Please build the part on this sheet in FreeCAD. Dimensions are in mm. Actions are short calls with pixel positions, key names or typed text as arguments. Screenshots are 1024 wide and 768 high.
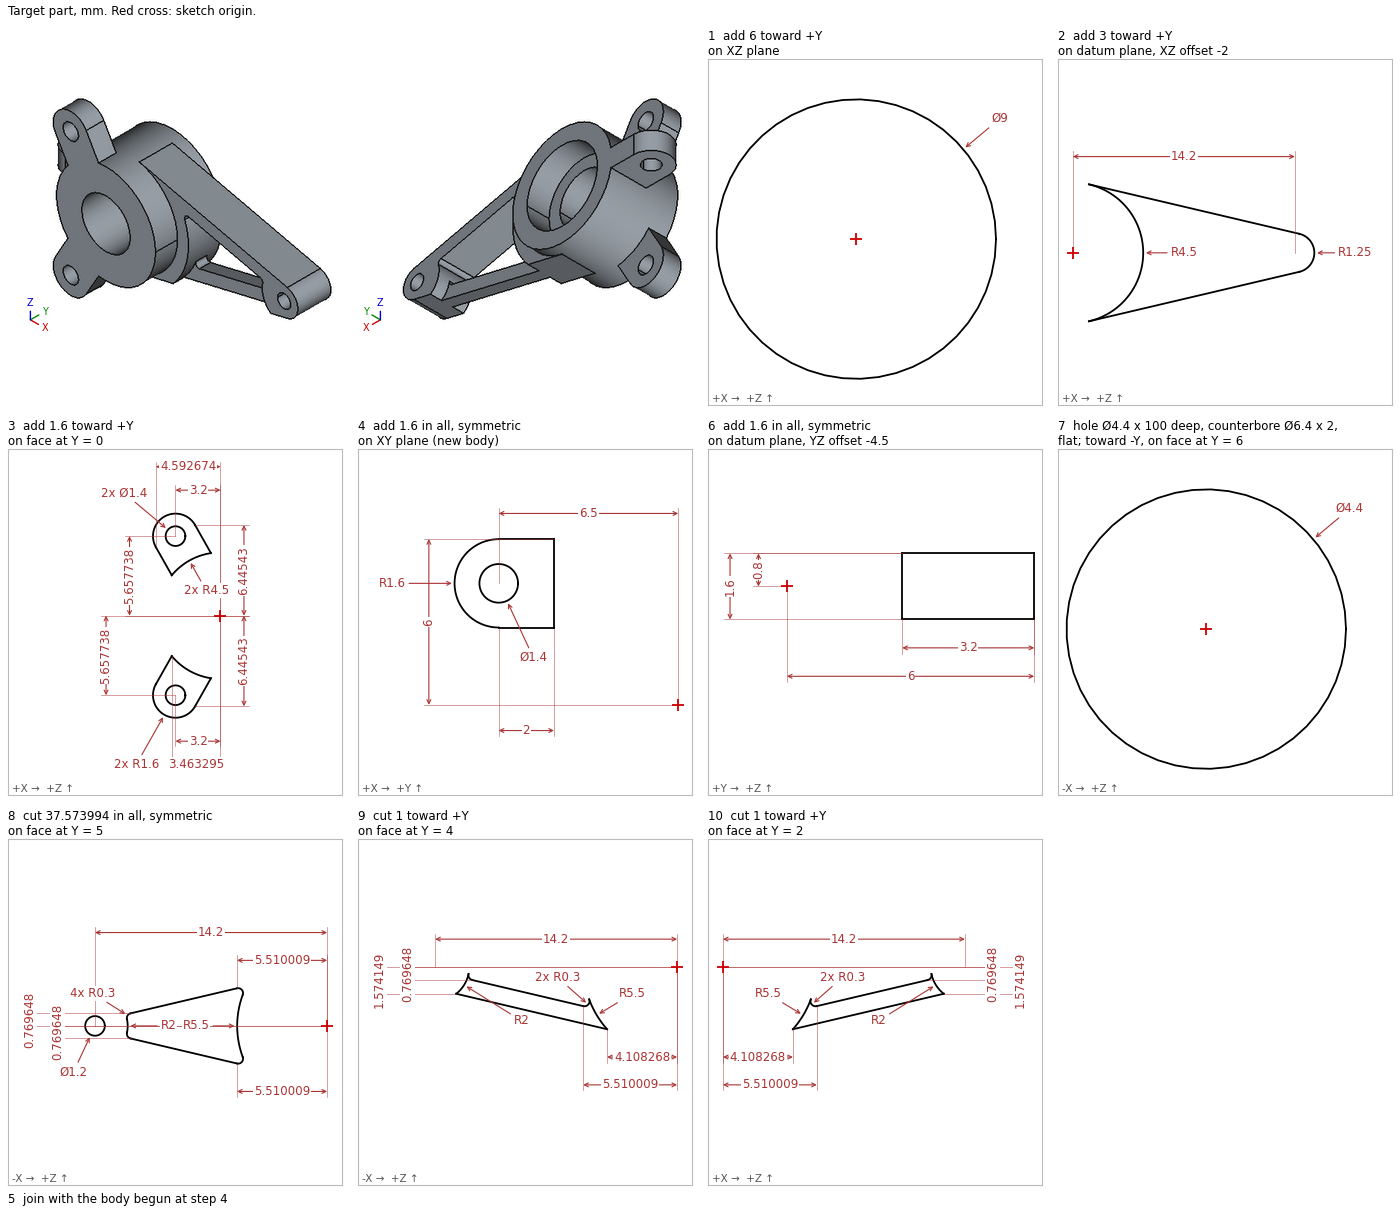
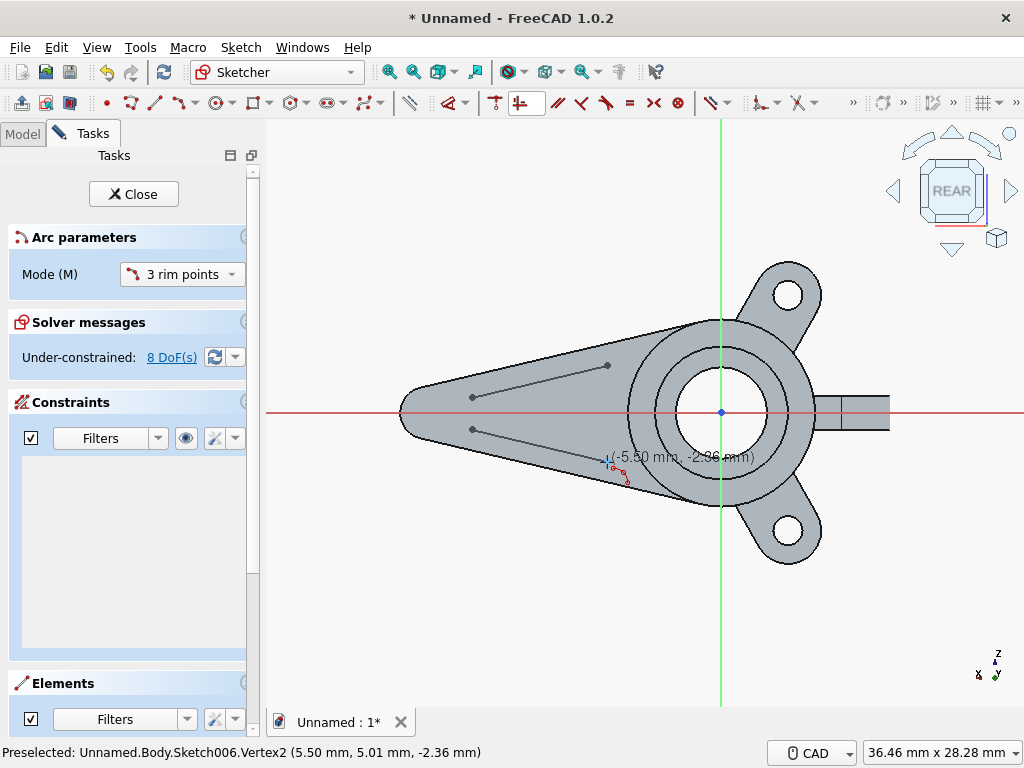
scroll(614, 453, up, 2)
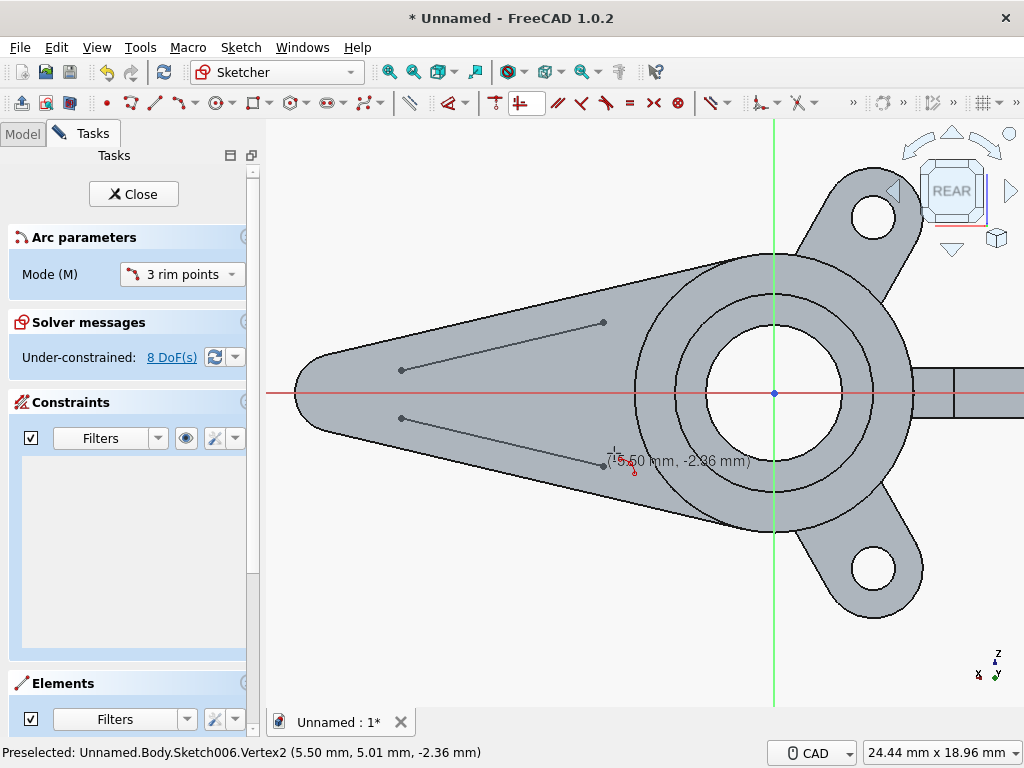
click(614, 452)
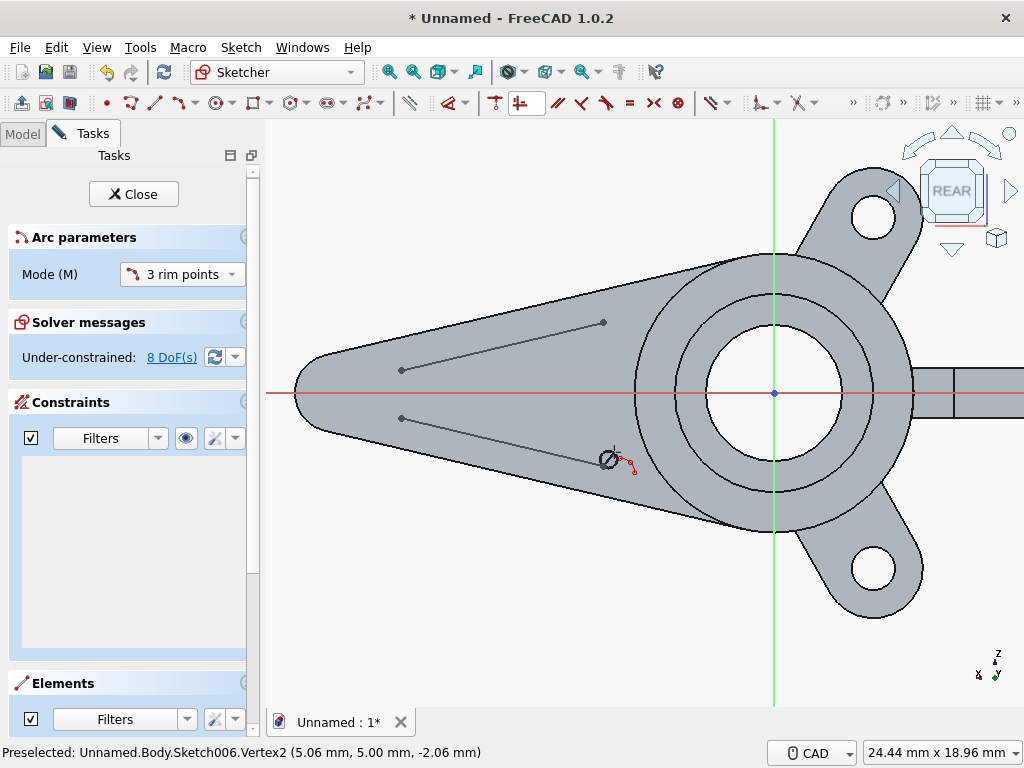
scroll(612, 461, up, 6)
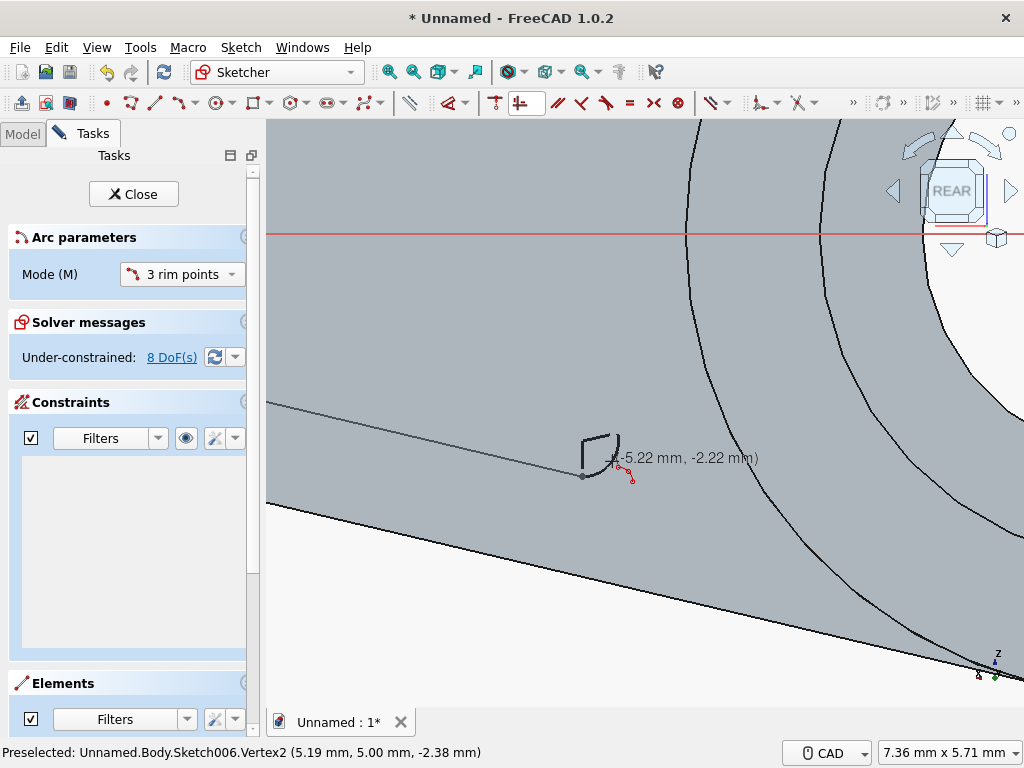
click(612, 461)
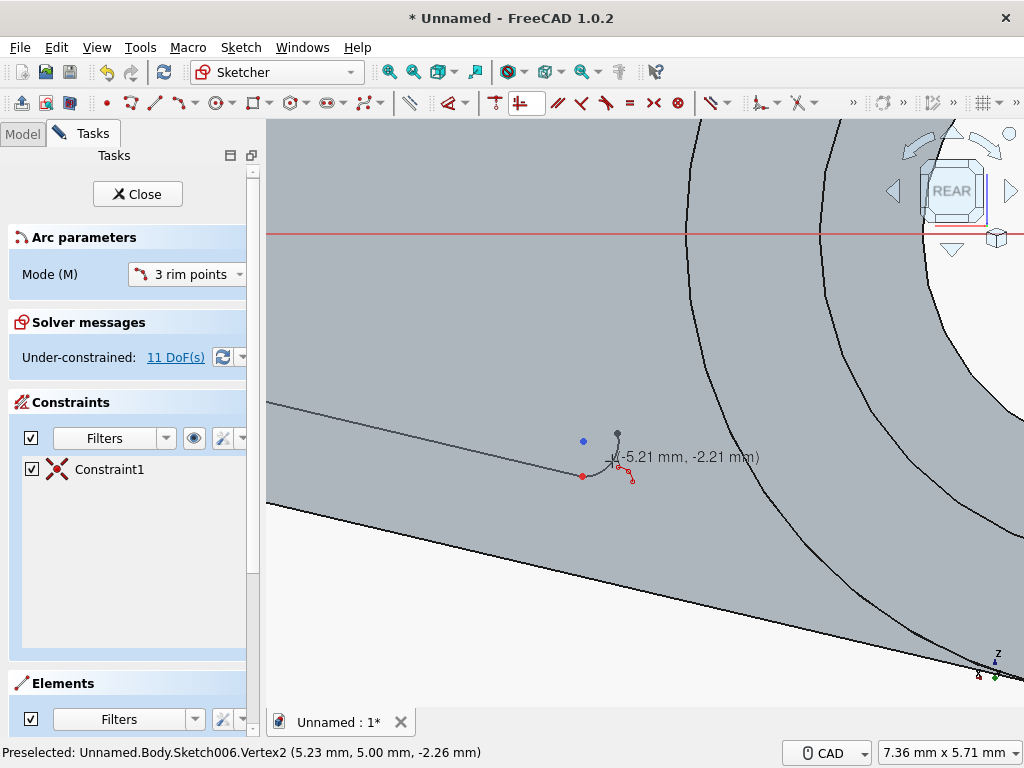
click(618, 433)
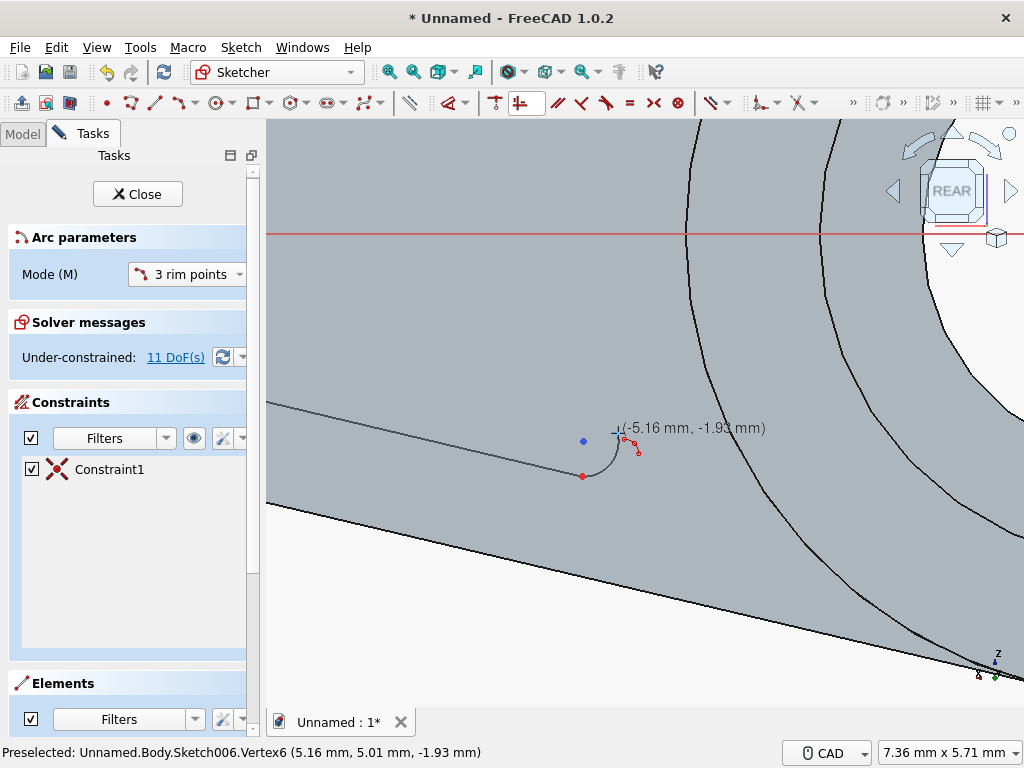
scroll(639, 472, down, 7)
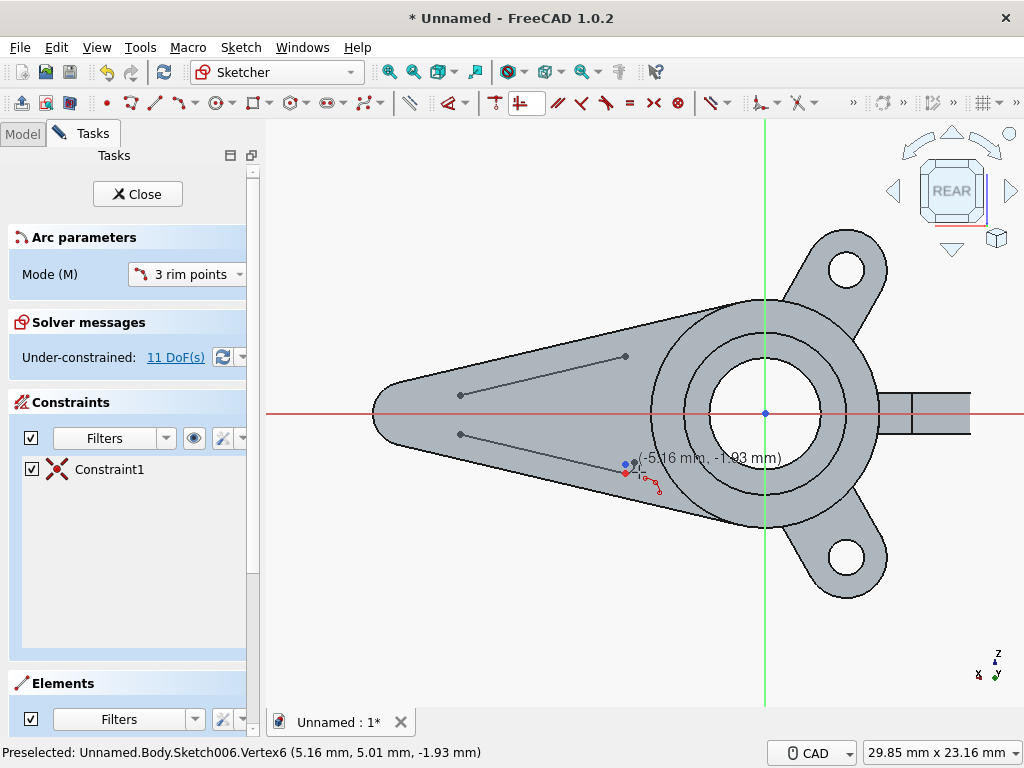
click(634, 365)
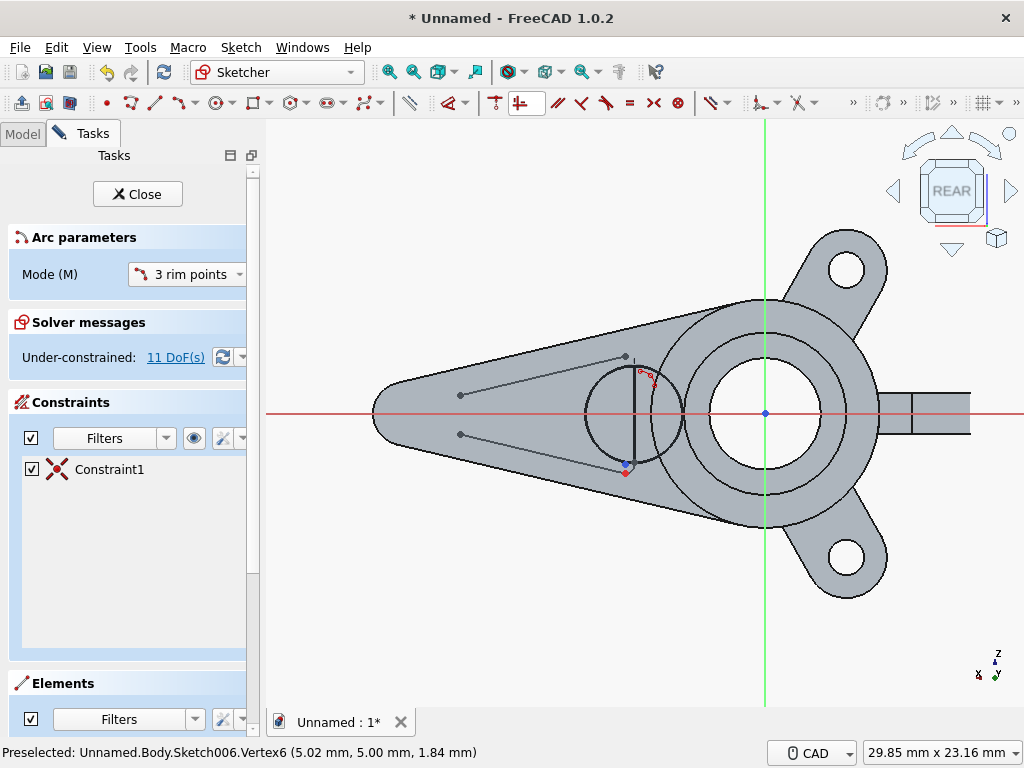
scroll(626, 404, up, 4)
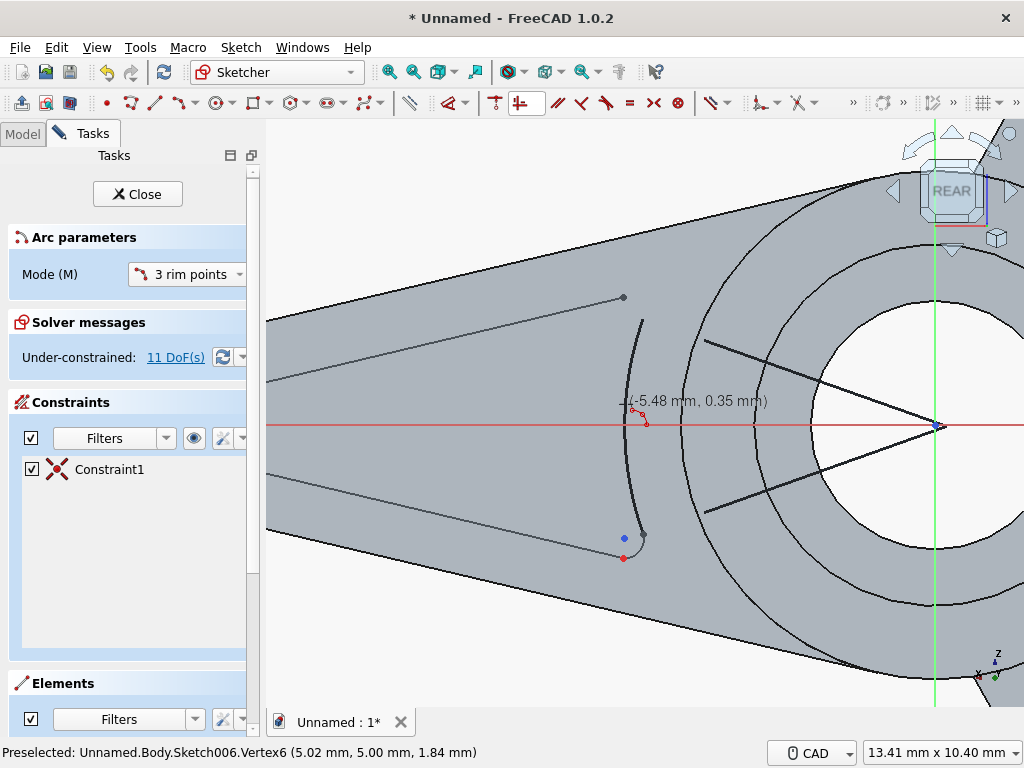
click(625, 403)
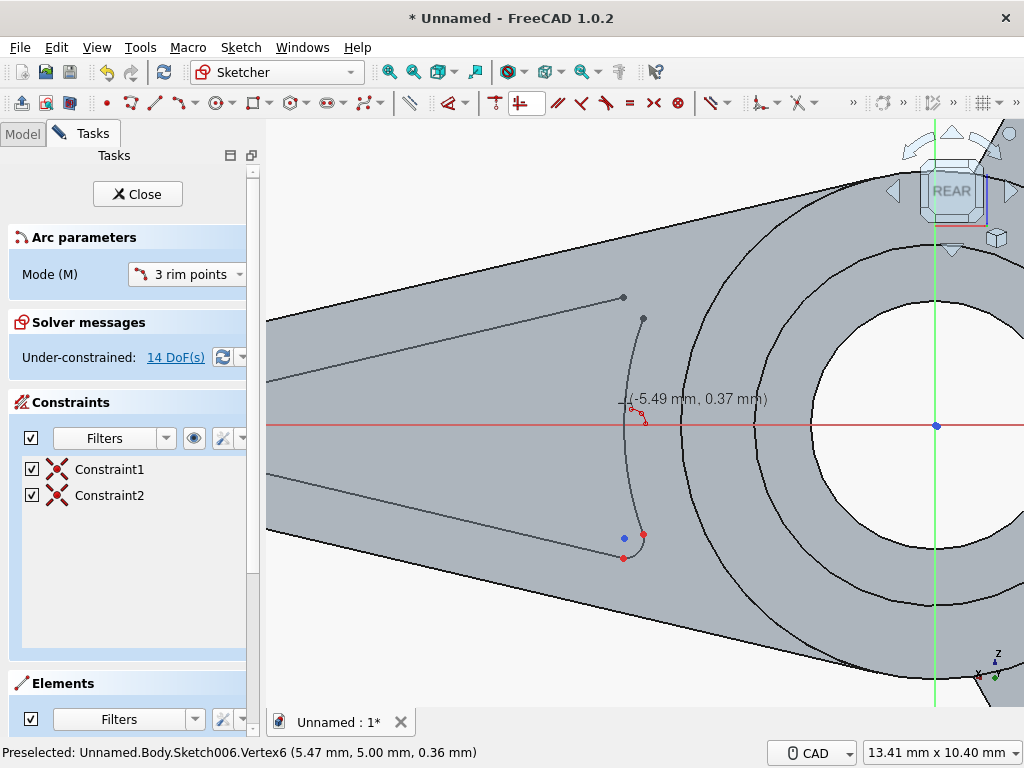
click(643, 319)
click(624, 297)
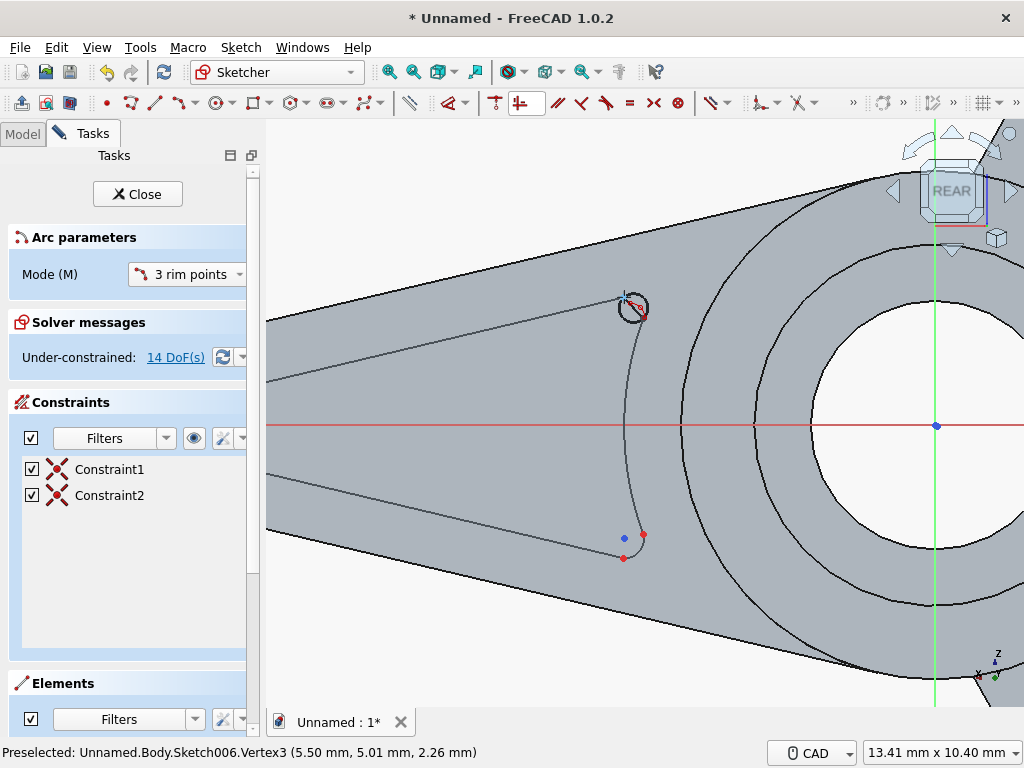
scroll(640, 300, up, 3)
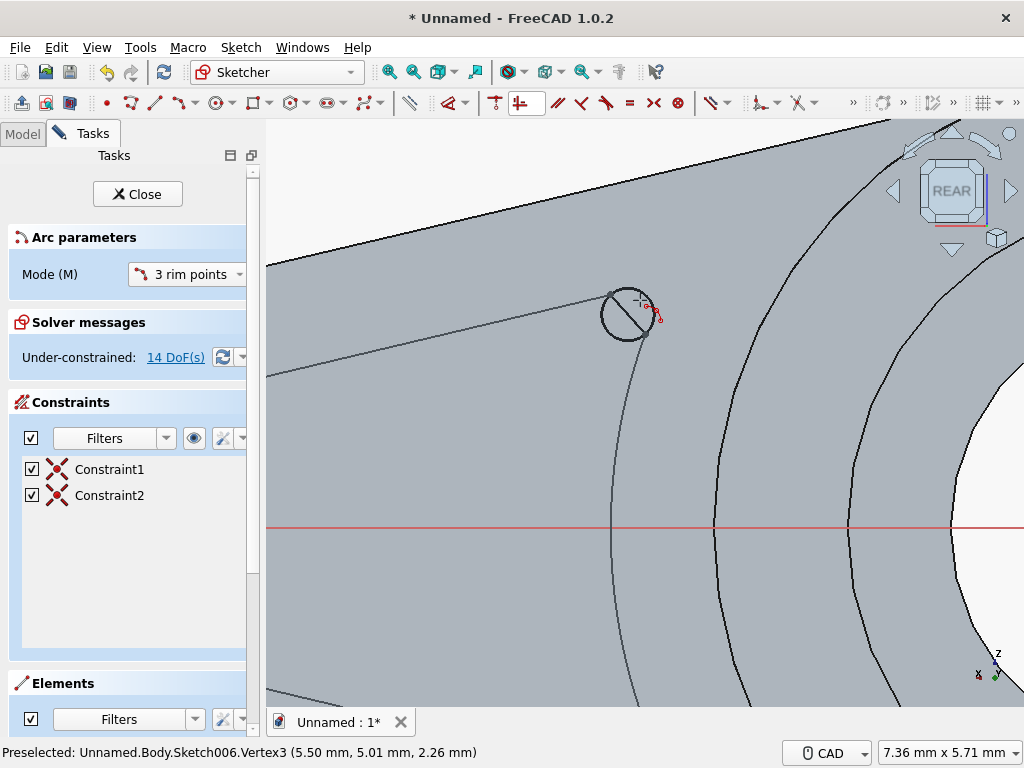
click(640, 301)